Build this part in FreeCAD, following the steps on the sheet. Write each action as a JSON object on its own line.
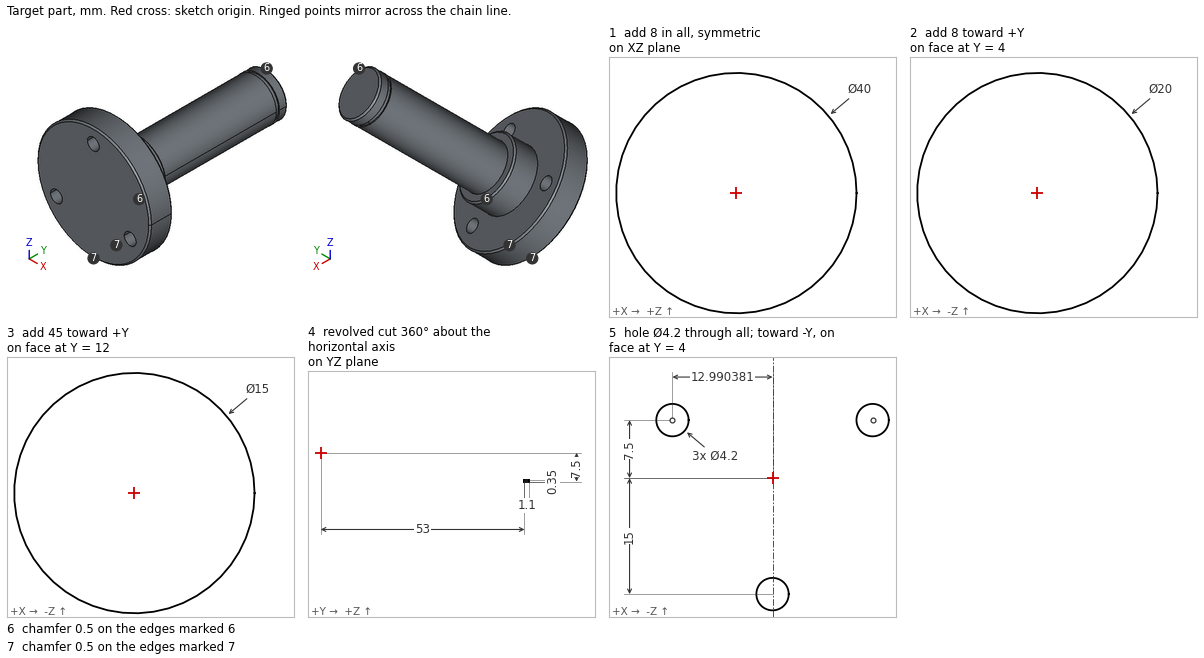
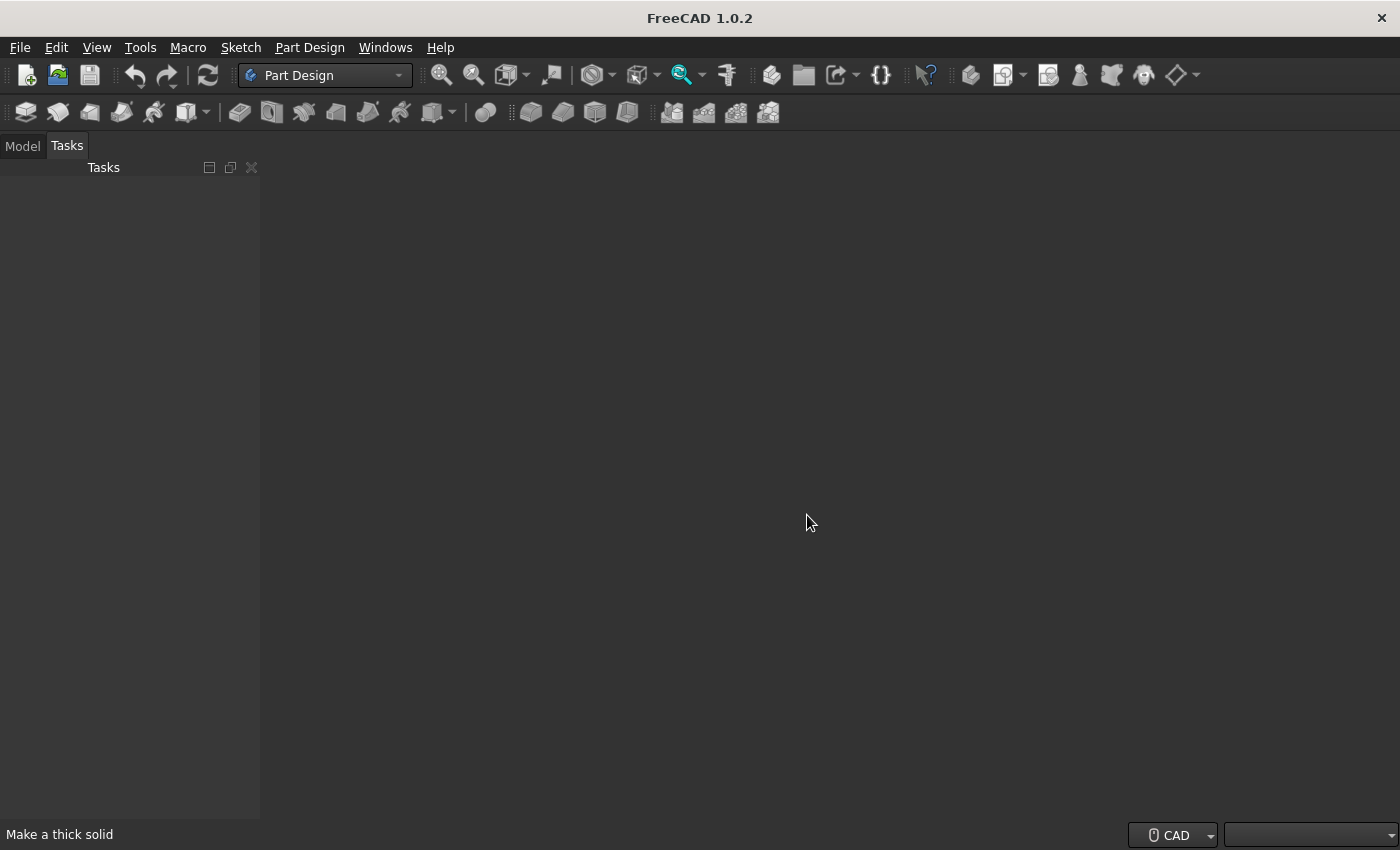
{"action": "left_click", "coordinate": [26, 76]}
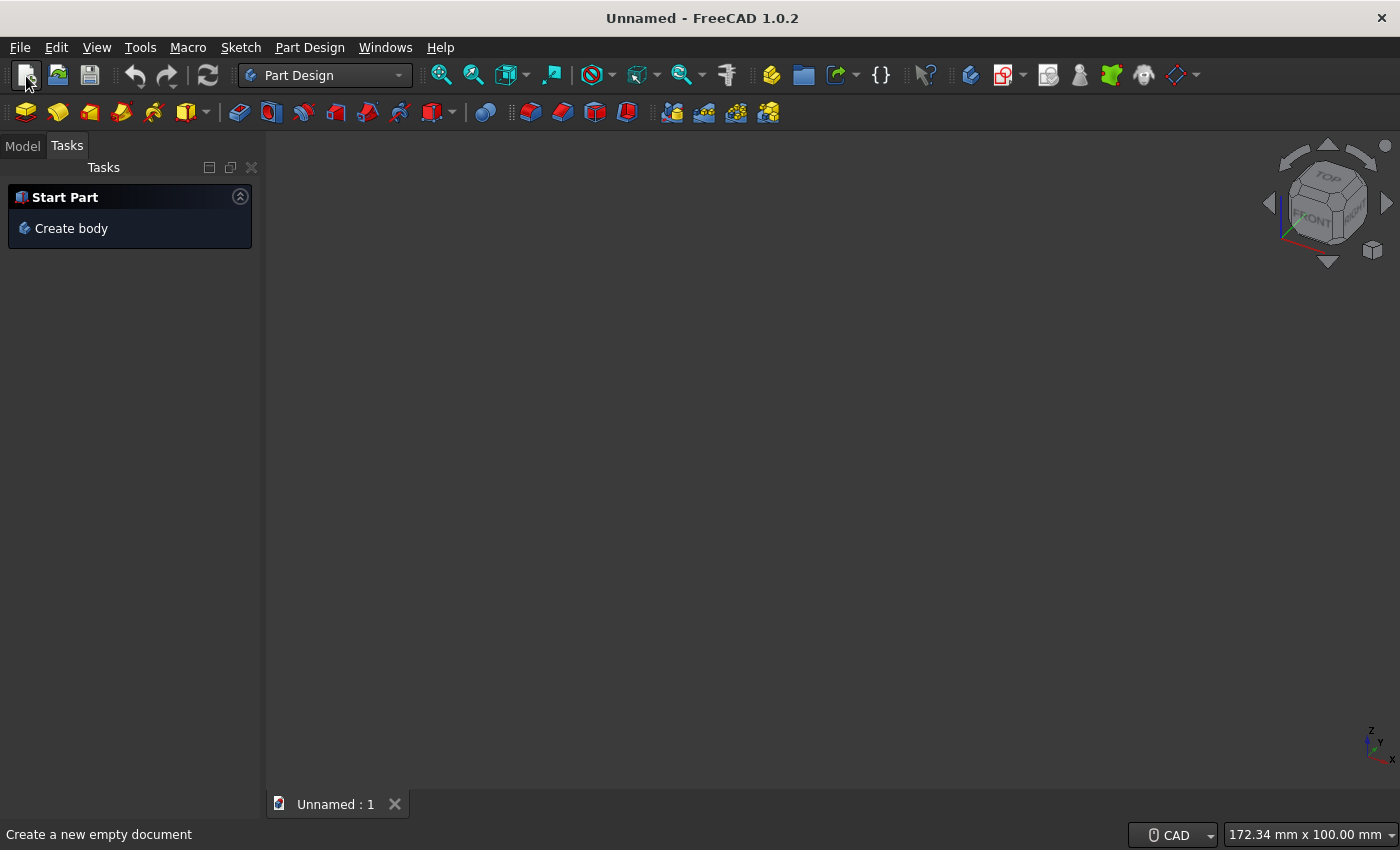
{"action": "left_click", "coordinate": [1004, 76]}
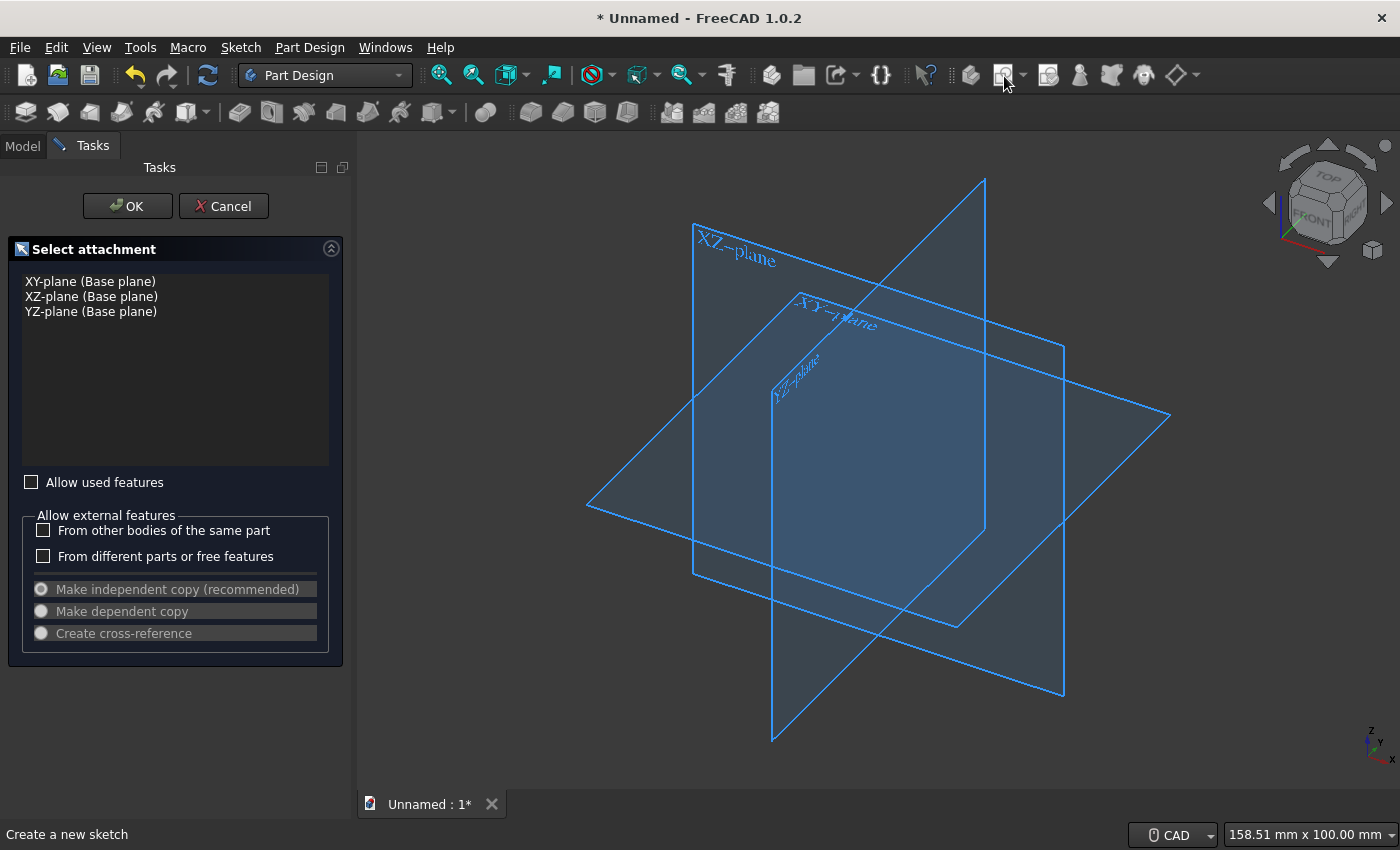
{"action": "left_click", "coordinate": [82, 296]}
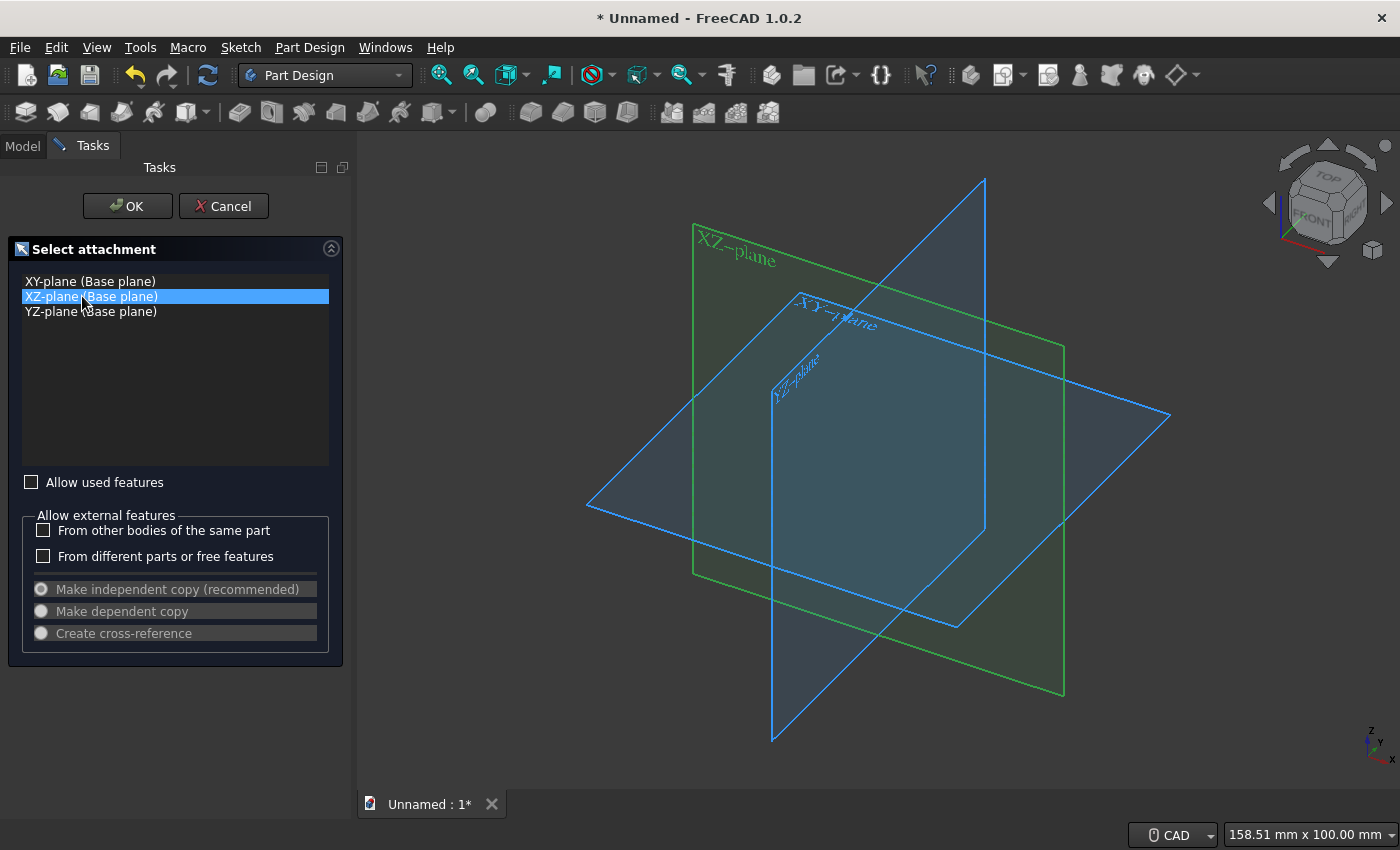
{"action": "left_click", "coordinate": [128, 206]}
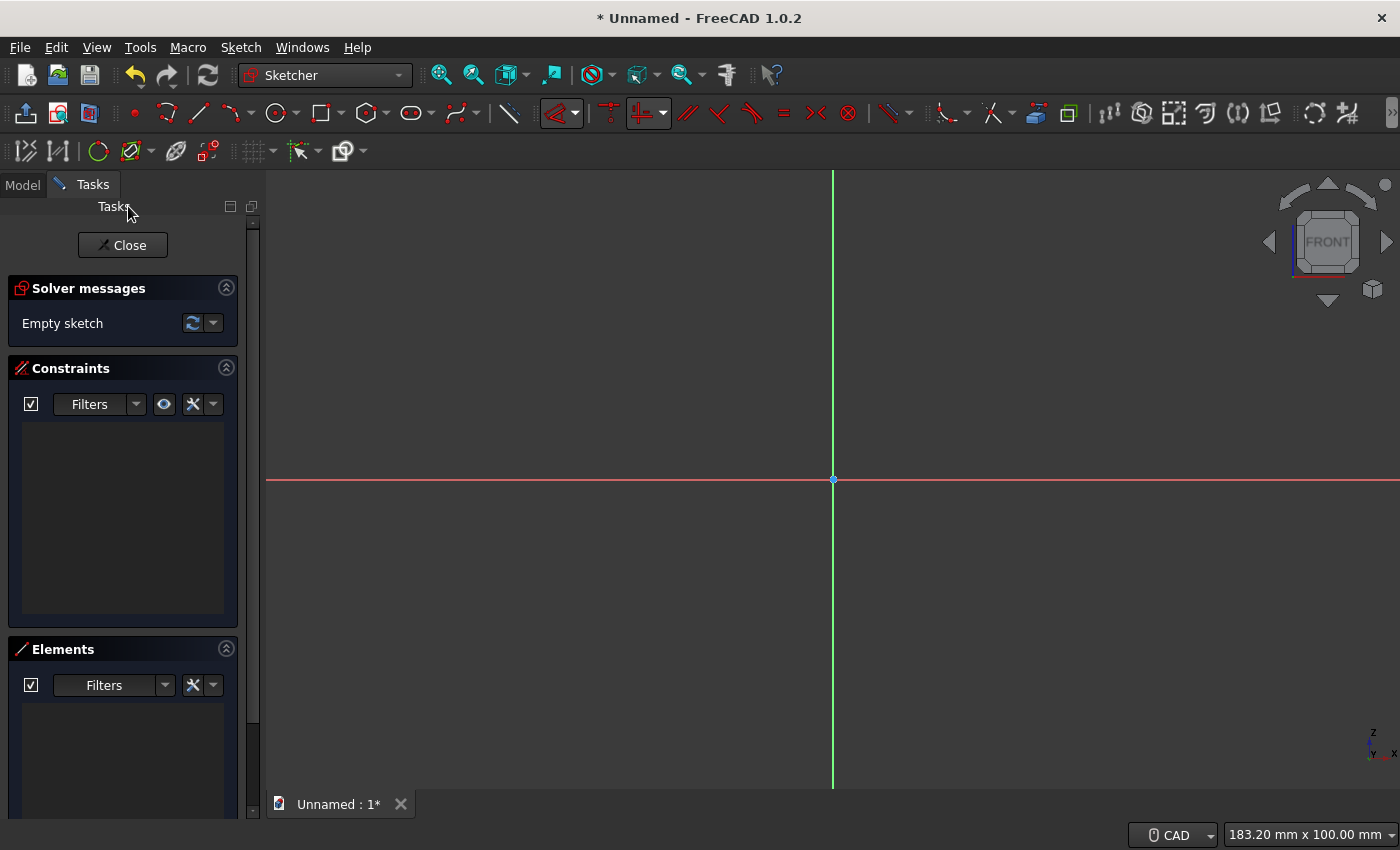
{"action": "scroll", "coordinate": [972, 480], "scroll_direction": "up", "scroll_amount": 2}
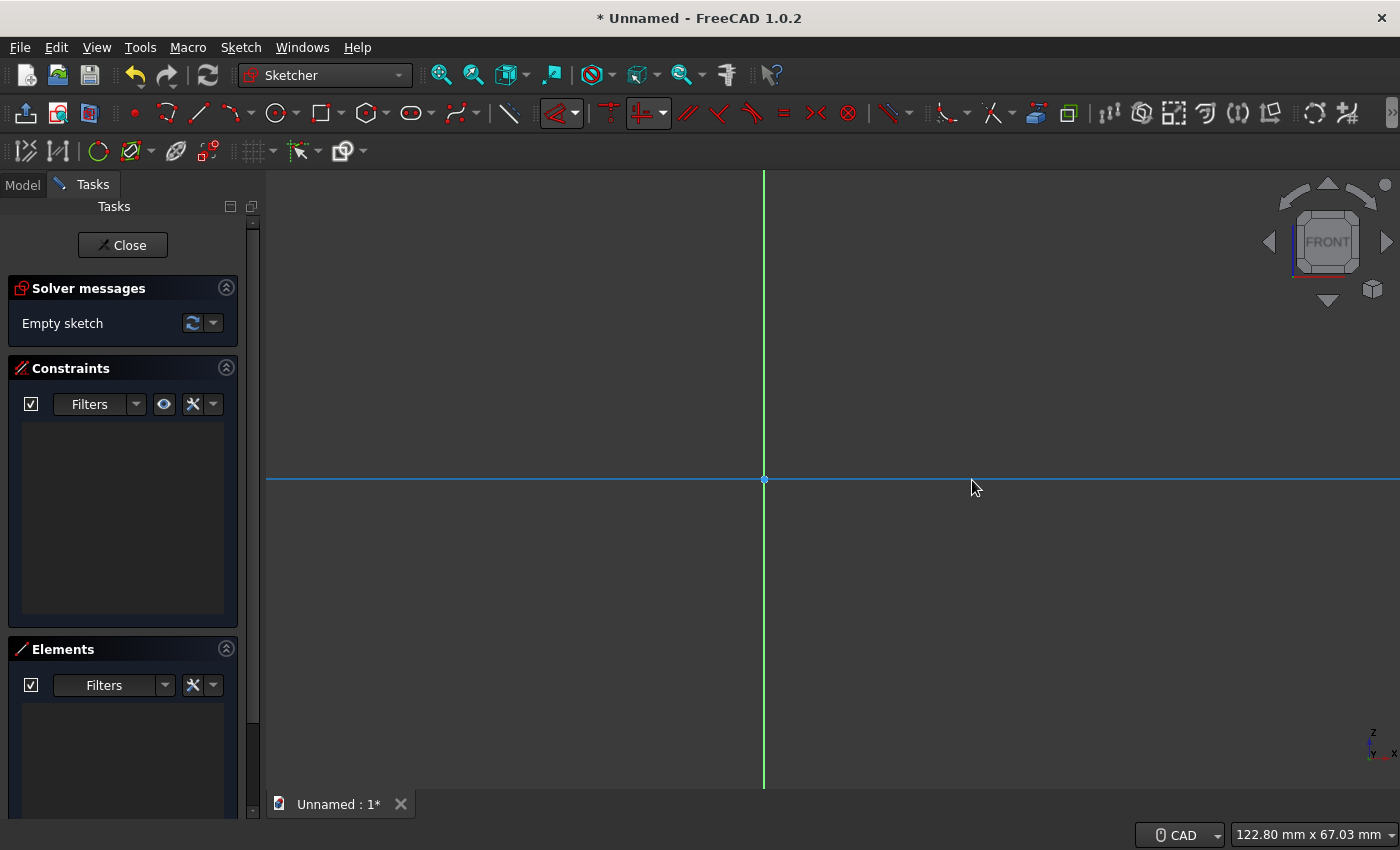
{"action": "left_click", "coordinate": [276, 114]}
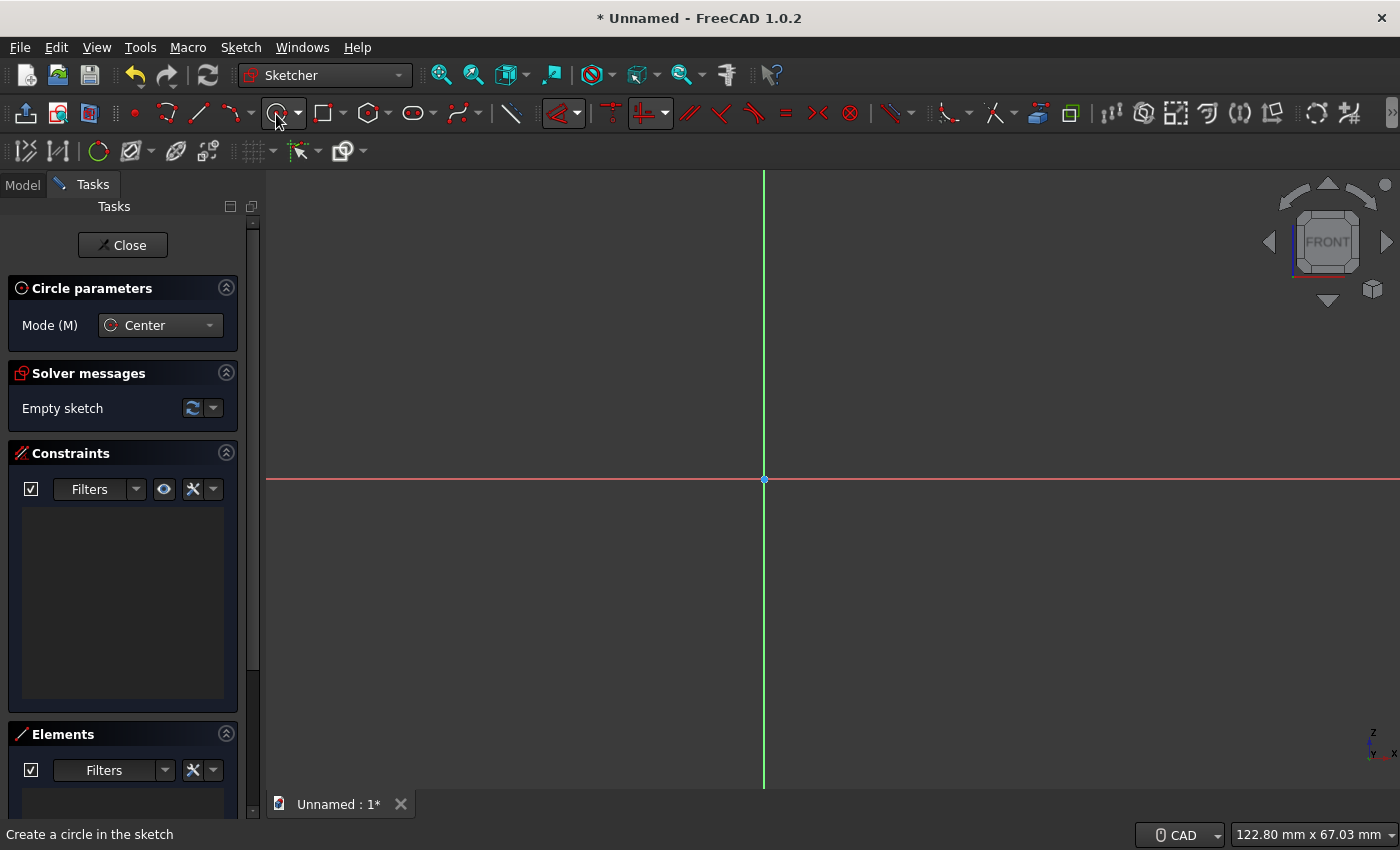
{"action": "left_click", "coordinate": [764, 479]}
{"action": "mouse_move", "coordinate": [895, 348]}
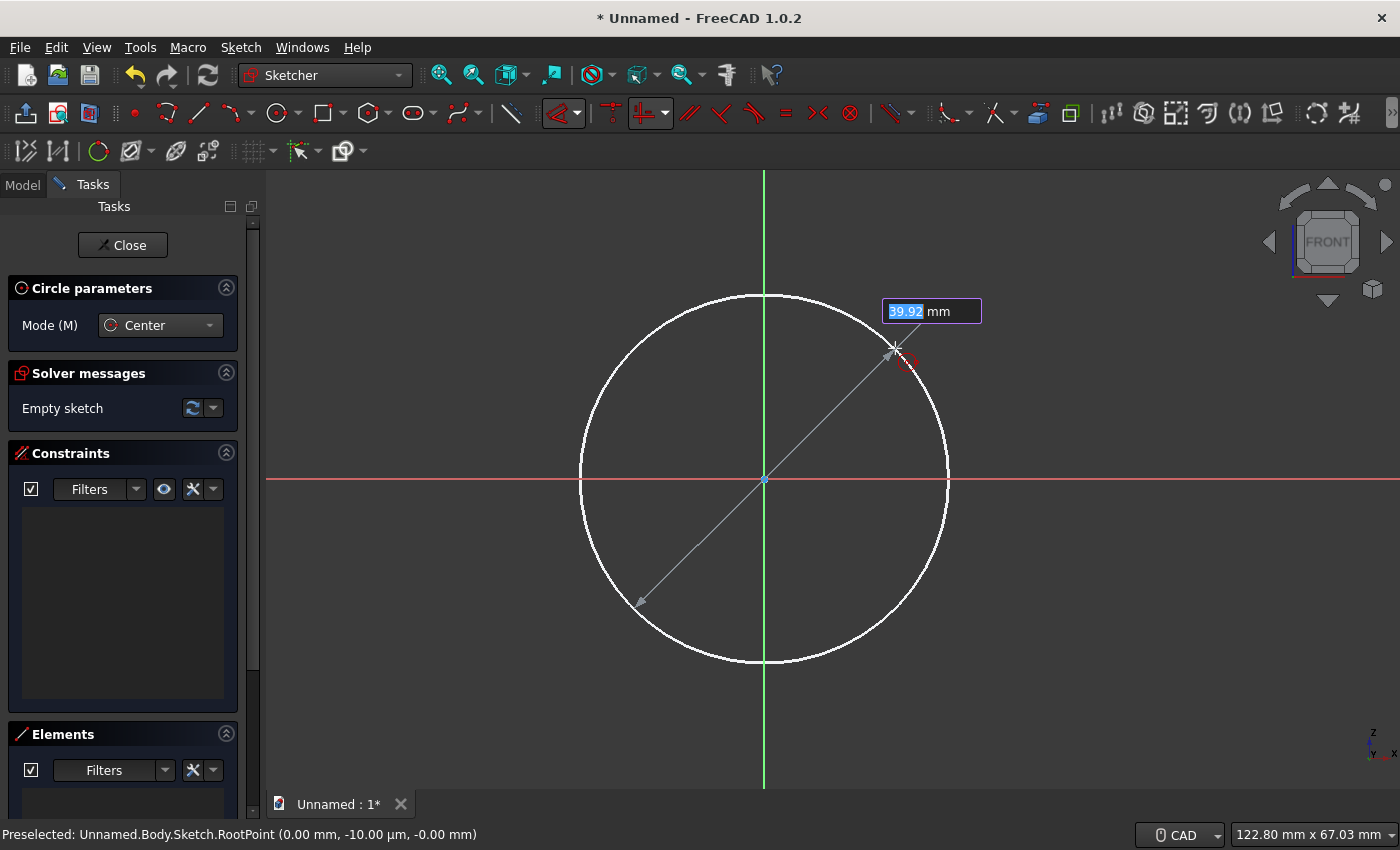
{"action": "type", "text": "40"}
{"action": "key", "text": "Return"}
{"action": "key", "text": "Escape"}